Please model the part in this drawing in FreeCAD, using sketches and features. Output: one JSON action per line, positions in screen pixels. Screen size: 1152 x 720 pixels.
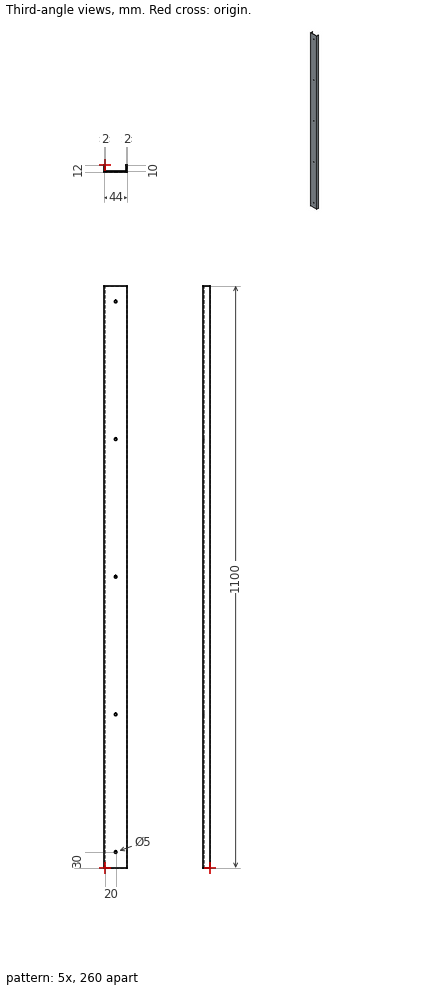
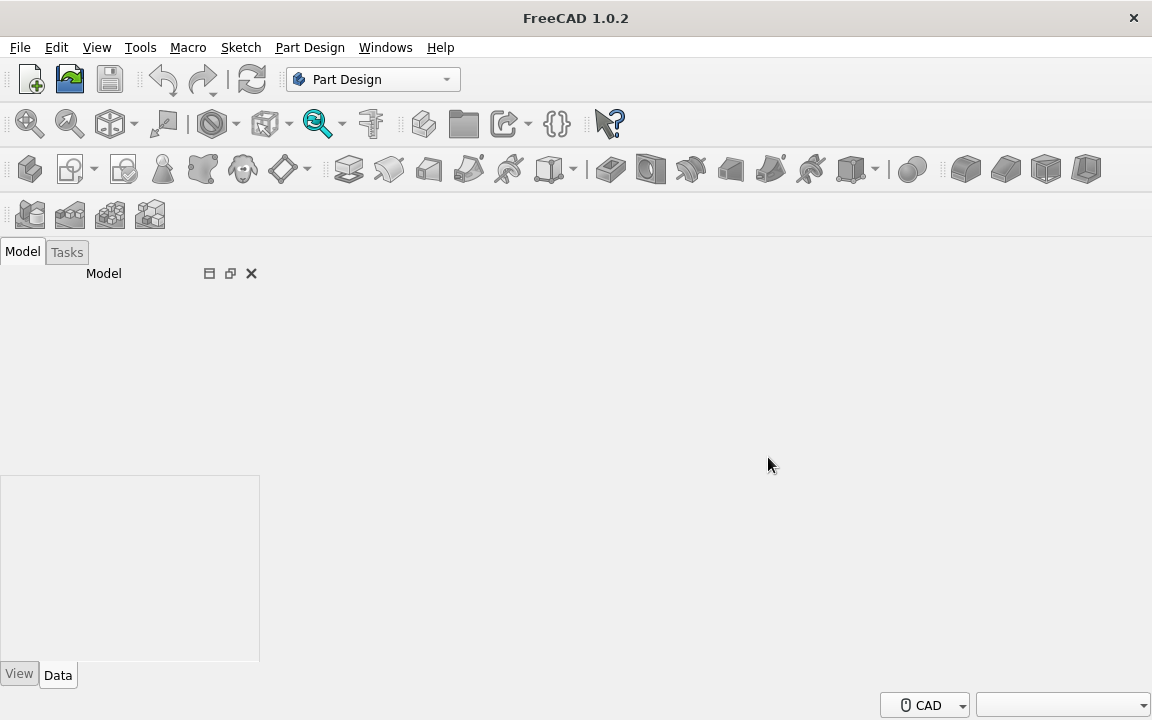
{"action": "left_click", "coordinate": [30, 80]}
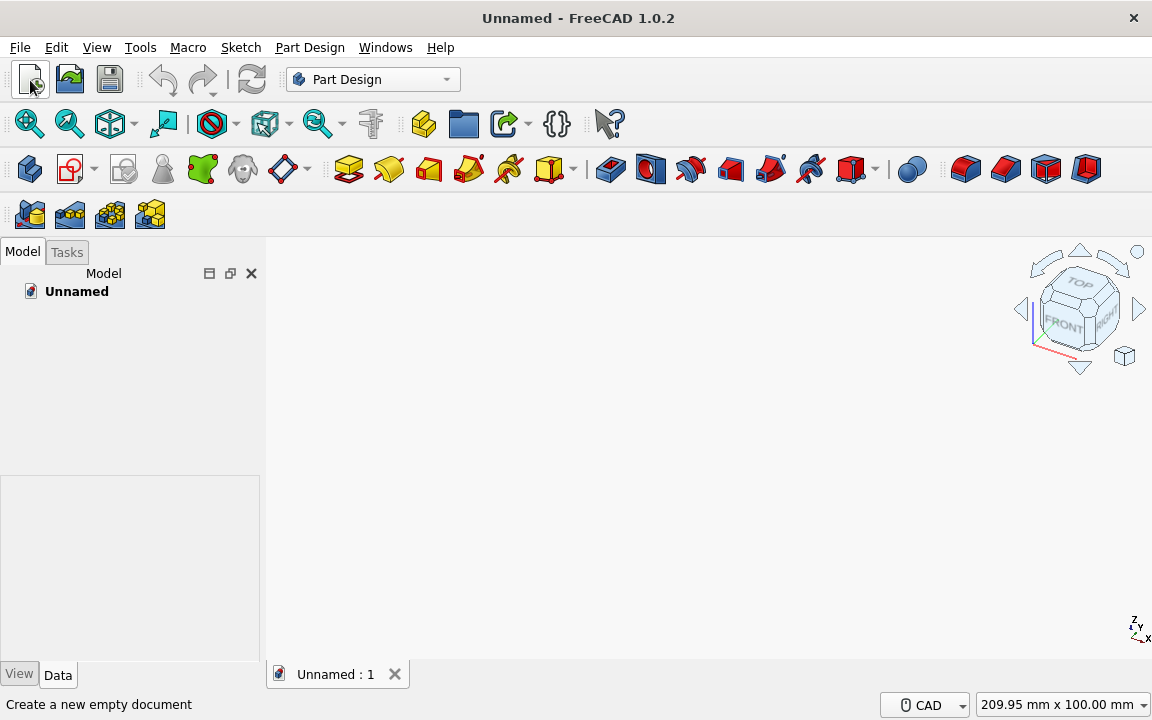
{"action": "left_click", "coordinate": [70, 170]}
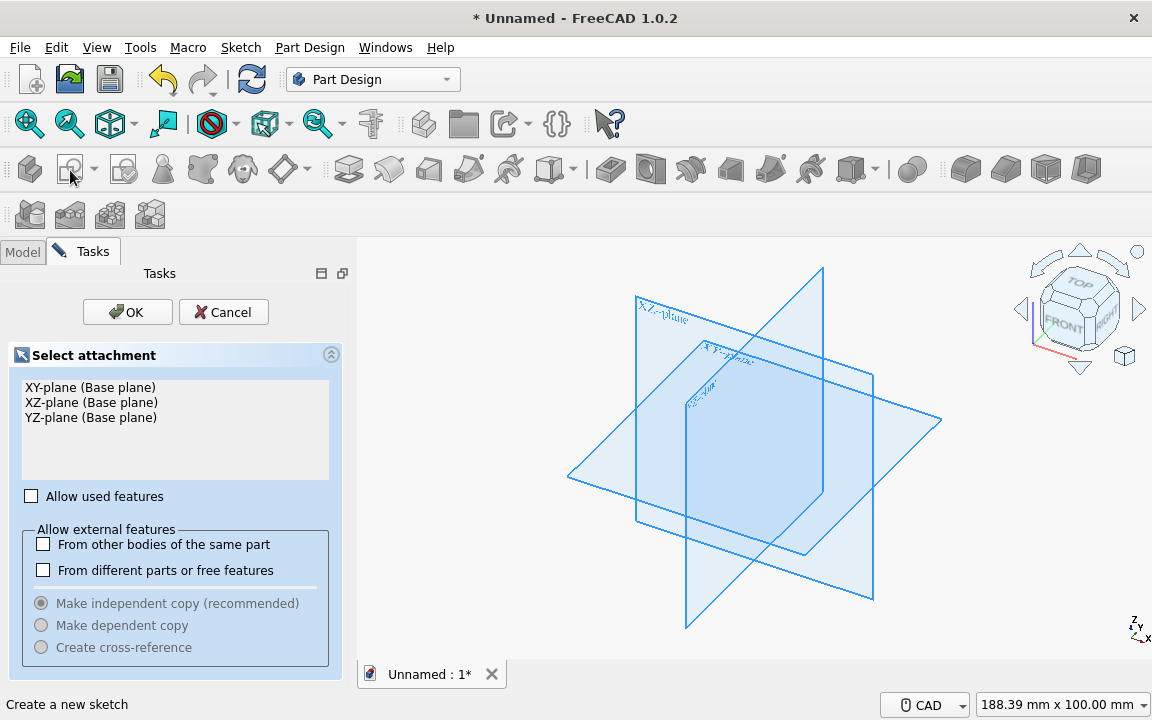
{"action": "left_click", "coordinate": [82, 388]}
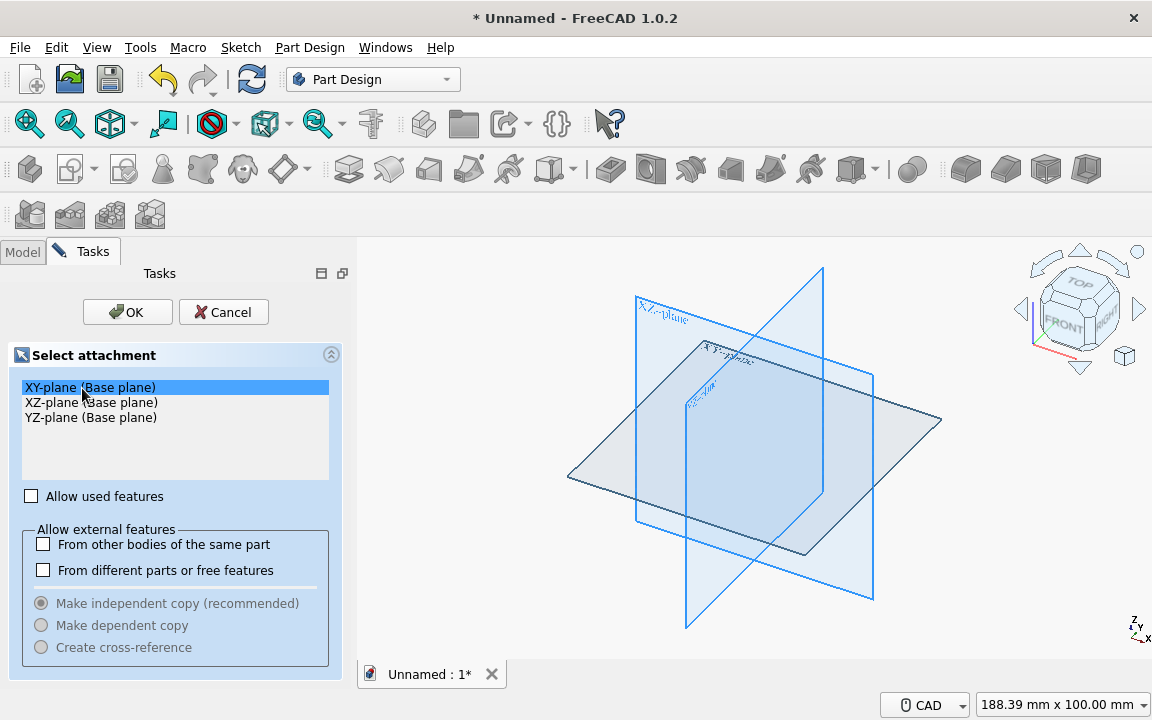
{"action": "left_click", "coordinate": [128, 312]}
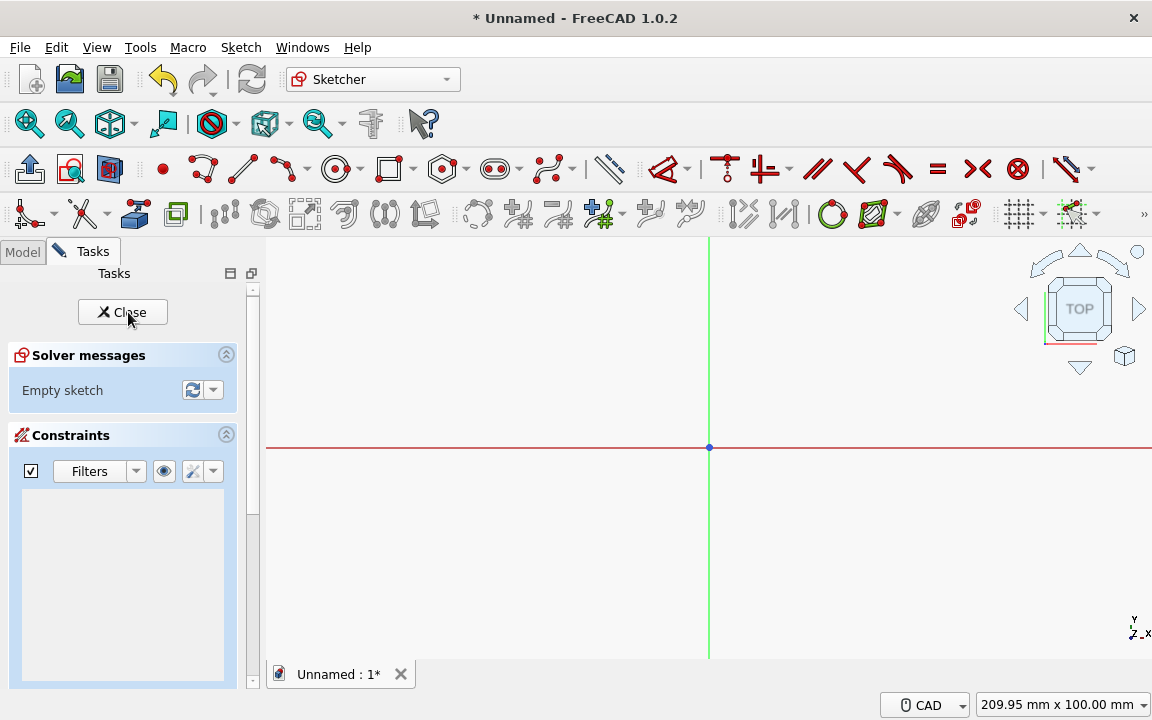
{"action": "scroll", "coordinate": [882, 488], "scroll_direction": "up", "scroll_amount": 5}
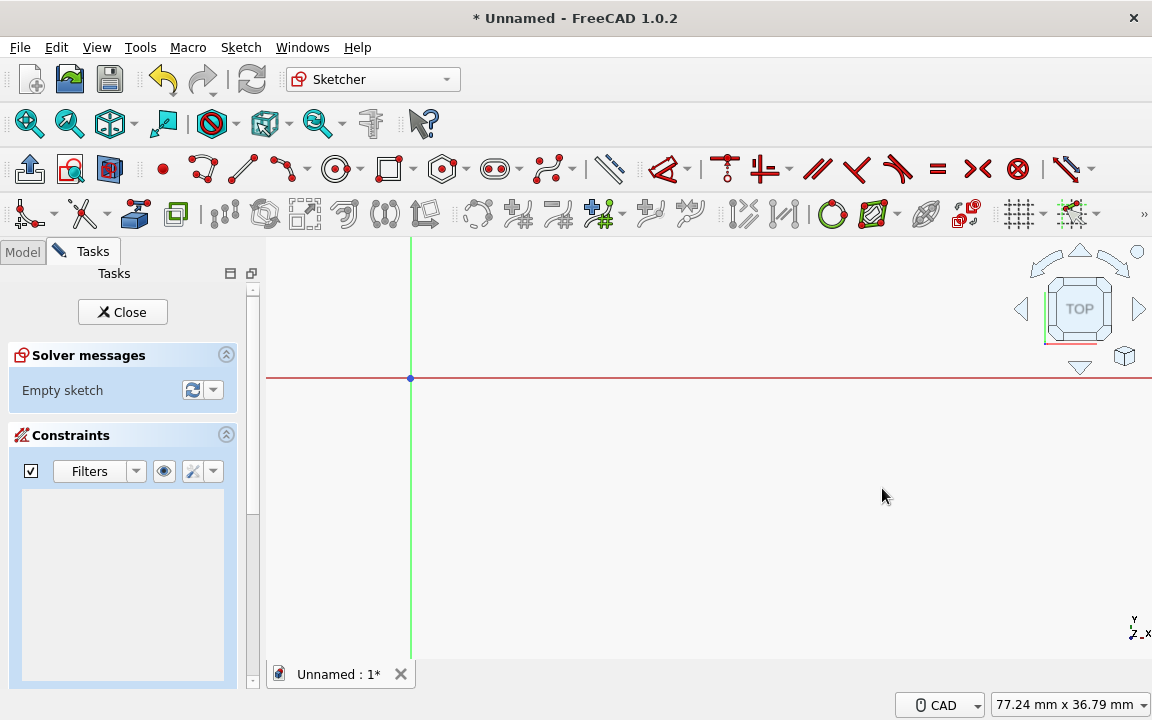
{"action": "left_click", "coordinate": [204, 170]}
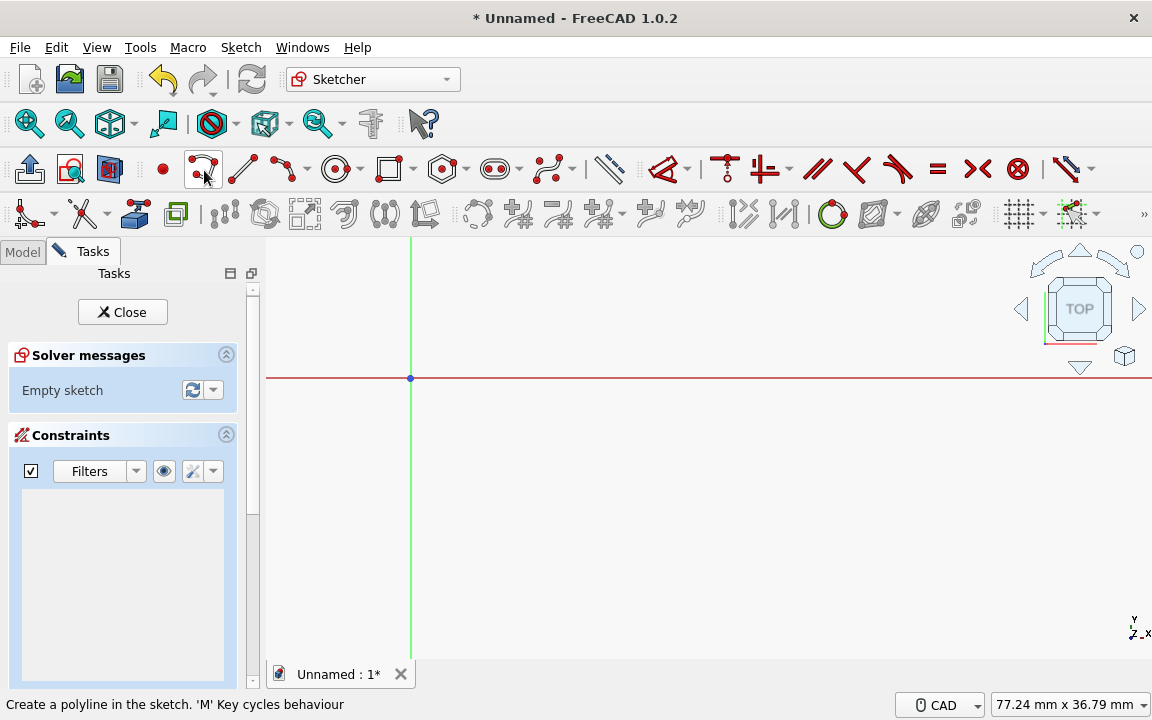
{"action": "left_click", "coordinate": [411, 378]}
{"action": "left_click", "coordinate": [388, 387]}
{"action": "left_click", "coordinate": [388, 516]}
{"action": "left_click", "coordinate": [892, 516]}
{"action": "left_click", "coordinate": [892, 378]}
{"action": "left_click", "coordinate": [869, 387]}
{"action": "left_click", "coordinate": [869, 493]}
{"action": "left_click", "coordinate": [420, 493]}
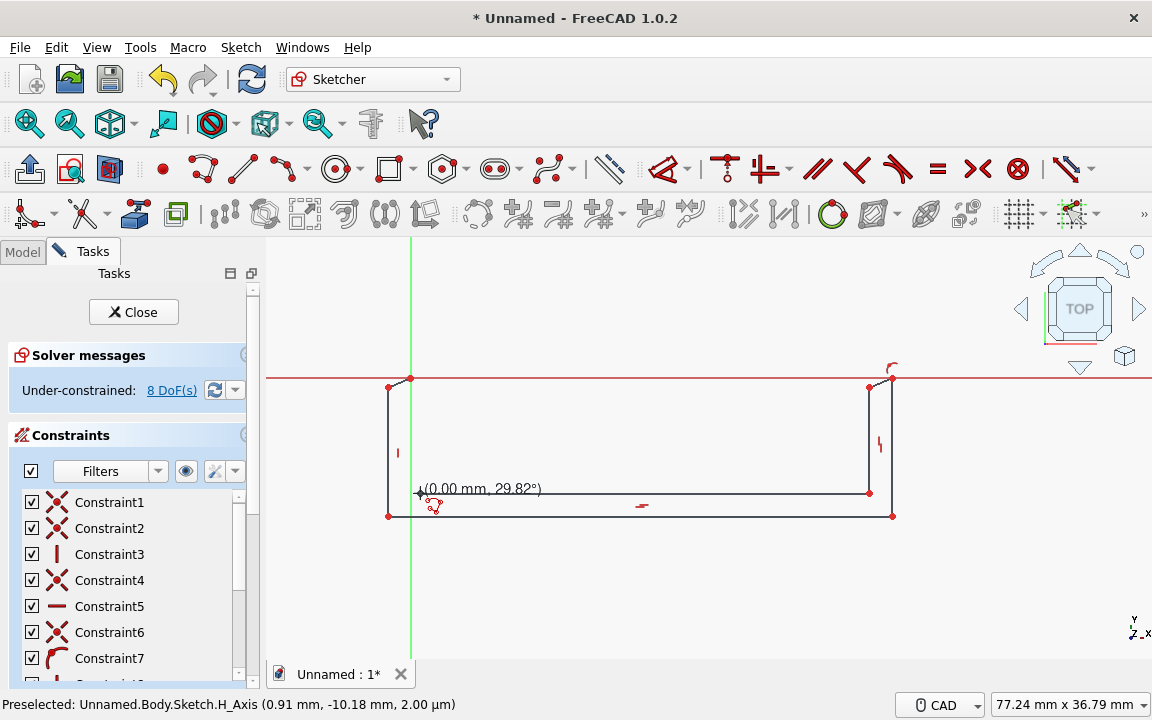
{"action": "scroll", "coordinate": [411, 378], "scroll_direction": "up", "scroll_amount": 2}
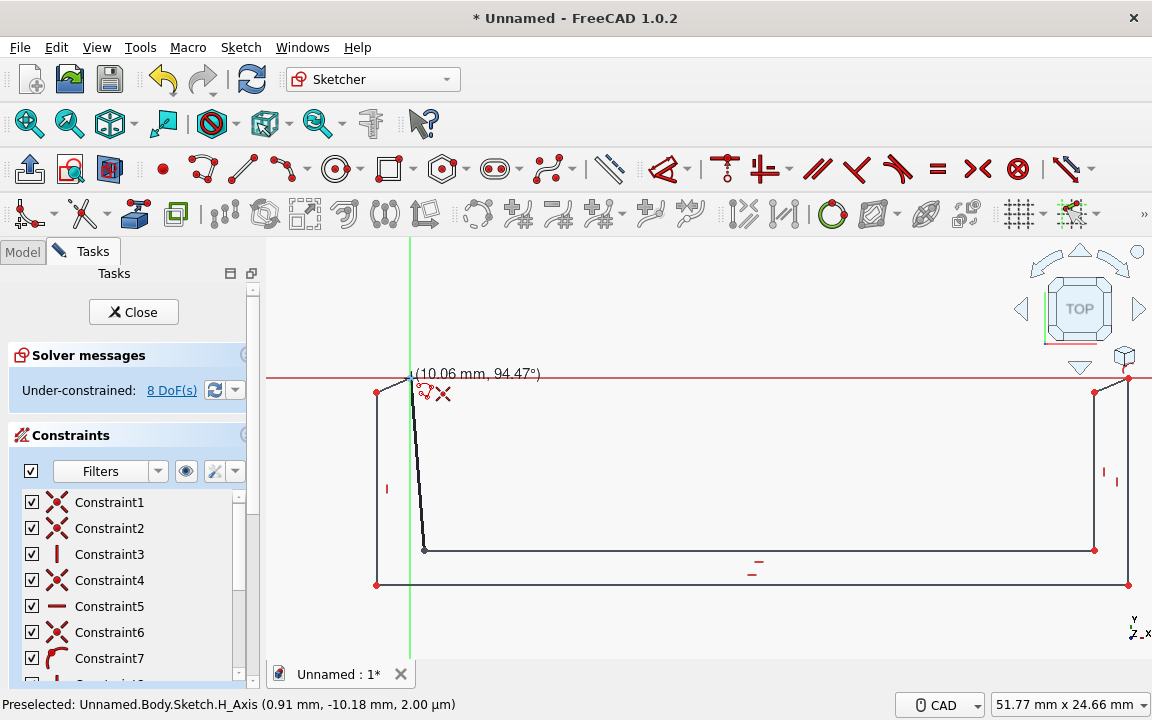
{"action": "left_click", "coordinate": [410, 378]}
{"action": "key", "text": "Escape"}
{"action": "key", "text": "Escape"}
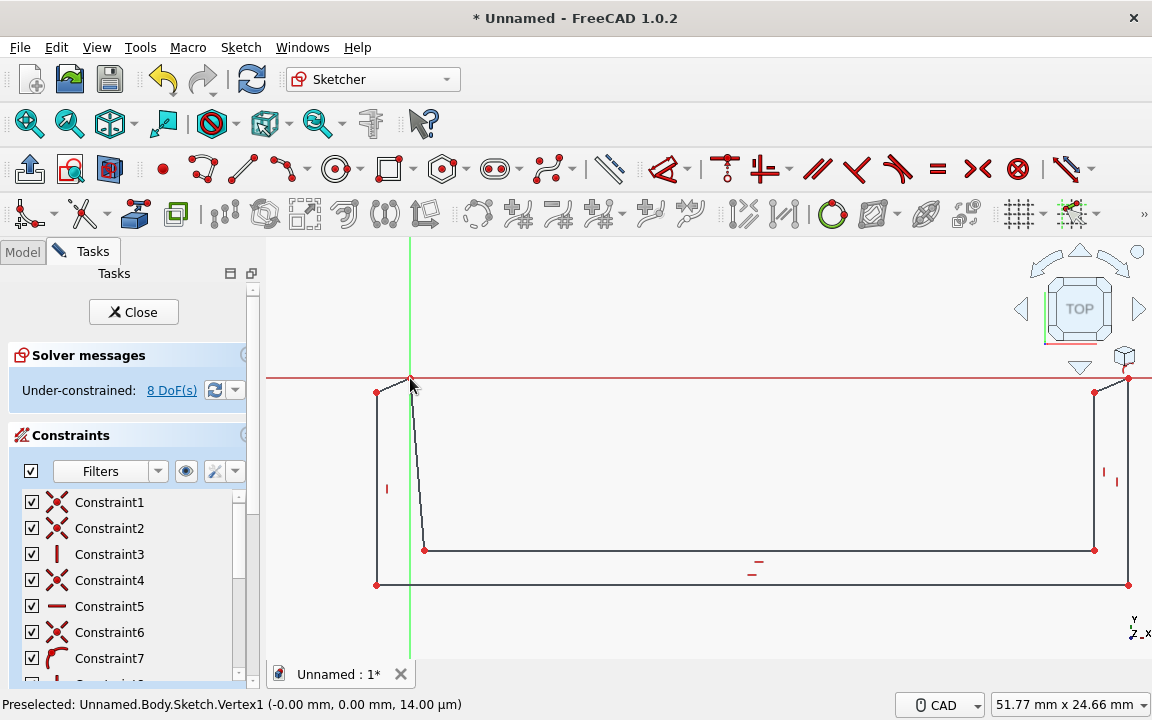
{"action": "scroll", "coordinate": [387, 388], "scroll_direction": "up", "scroll_amount": 2}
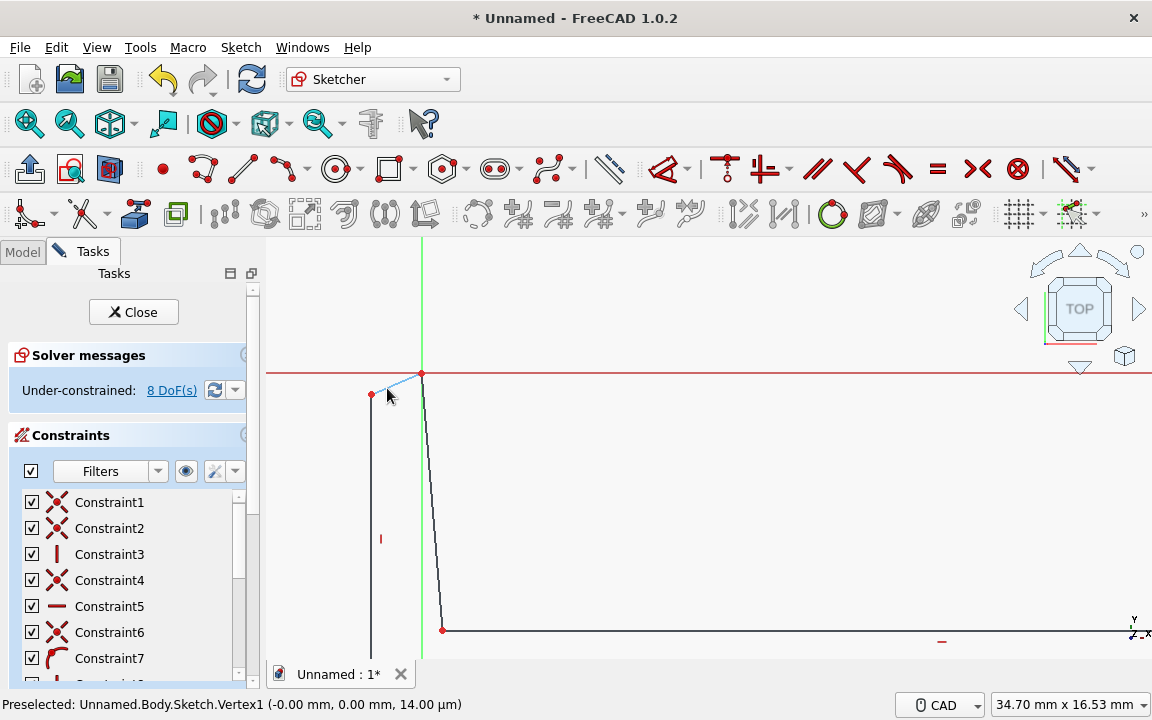
{"action": "left_click", "coordinate": [386, 388]}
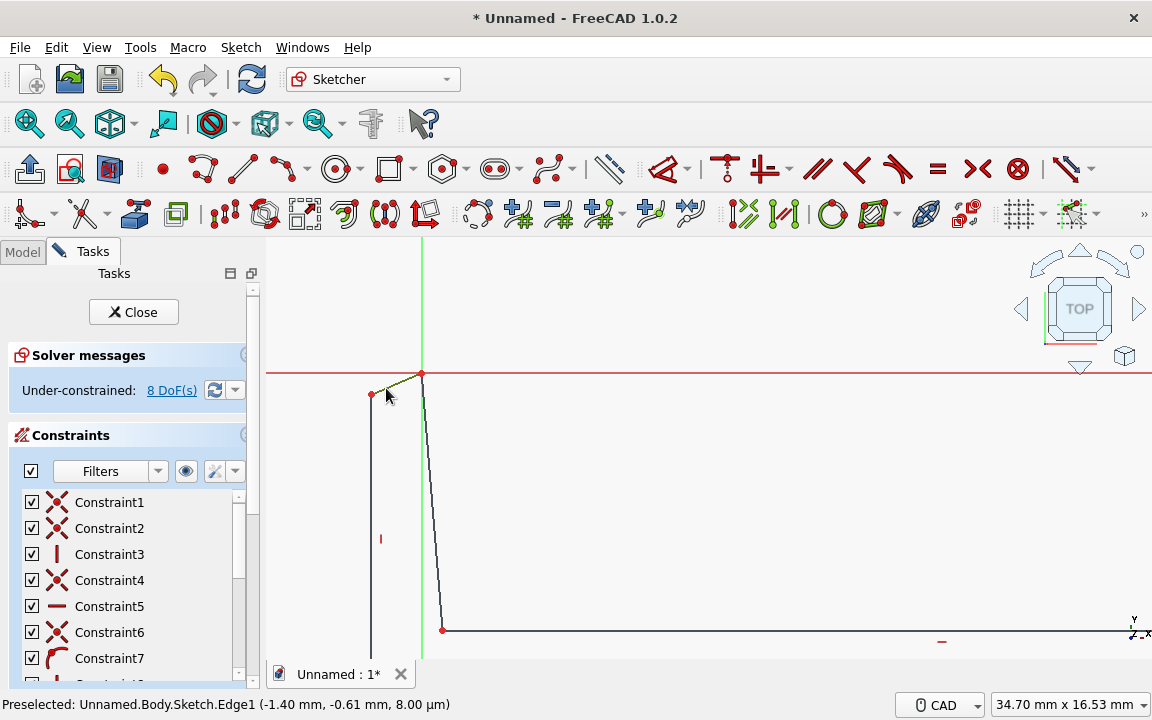
{"action": "key", "text": "h"}